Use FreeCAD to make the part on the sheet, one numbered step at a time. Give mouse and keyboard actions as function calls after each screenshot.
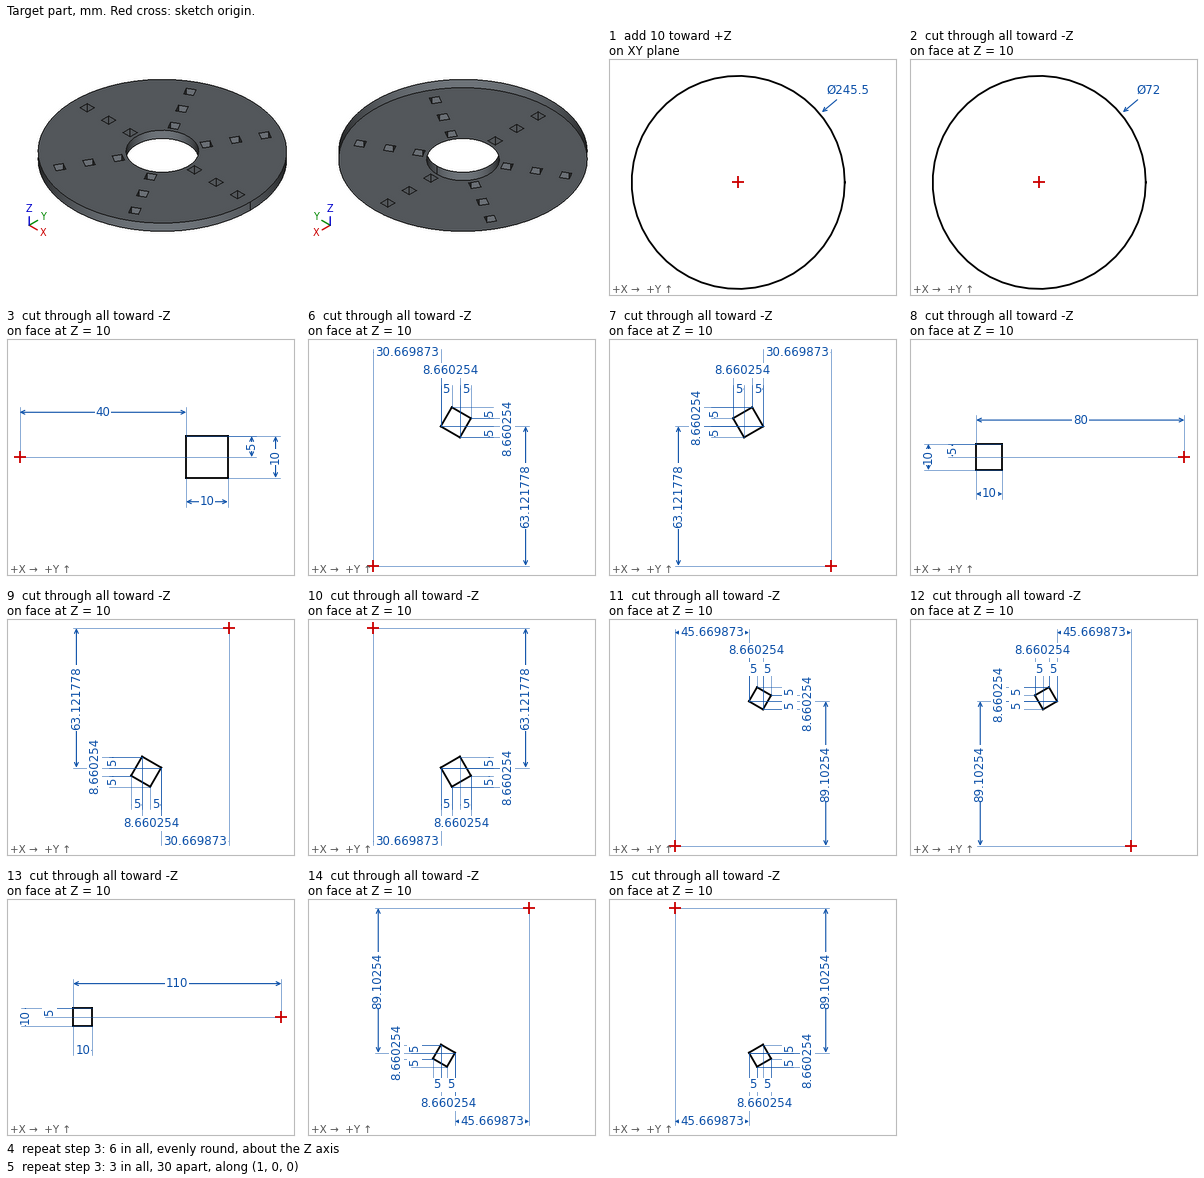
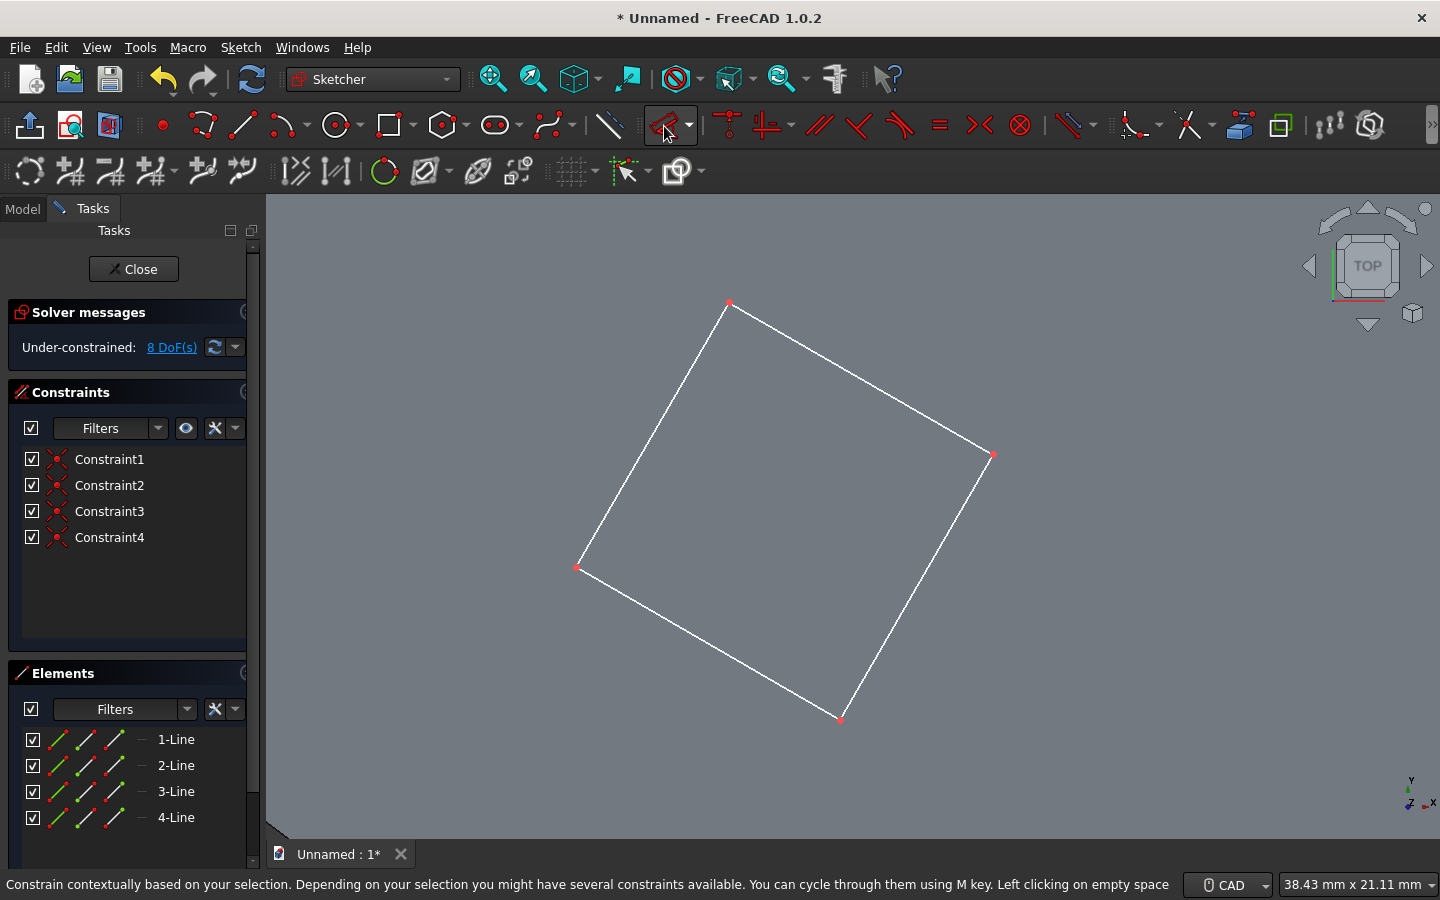
click(914, 409)
click(1027, 379)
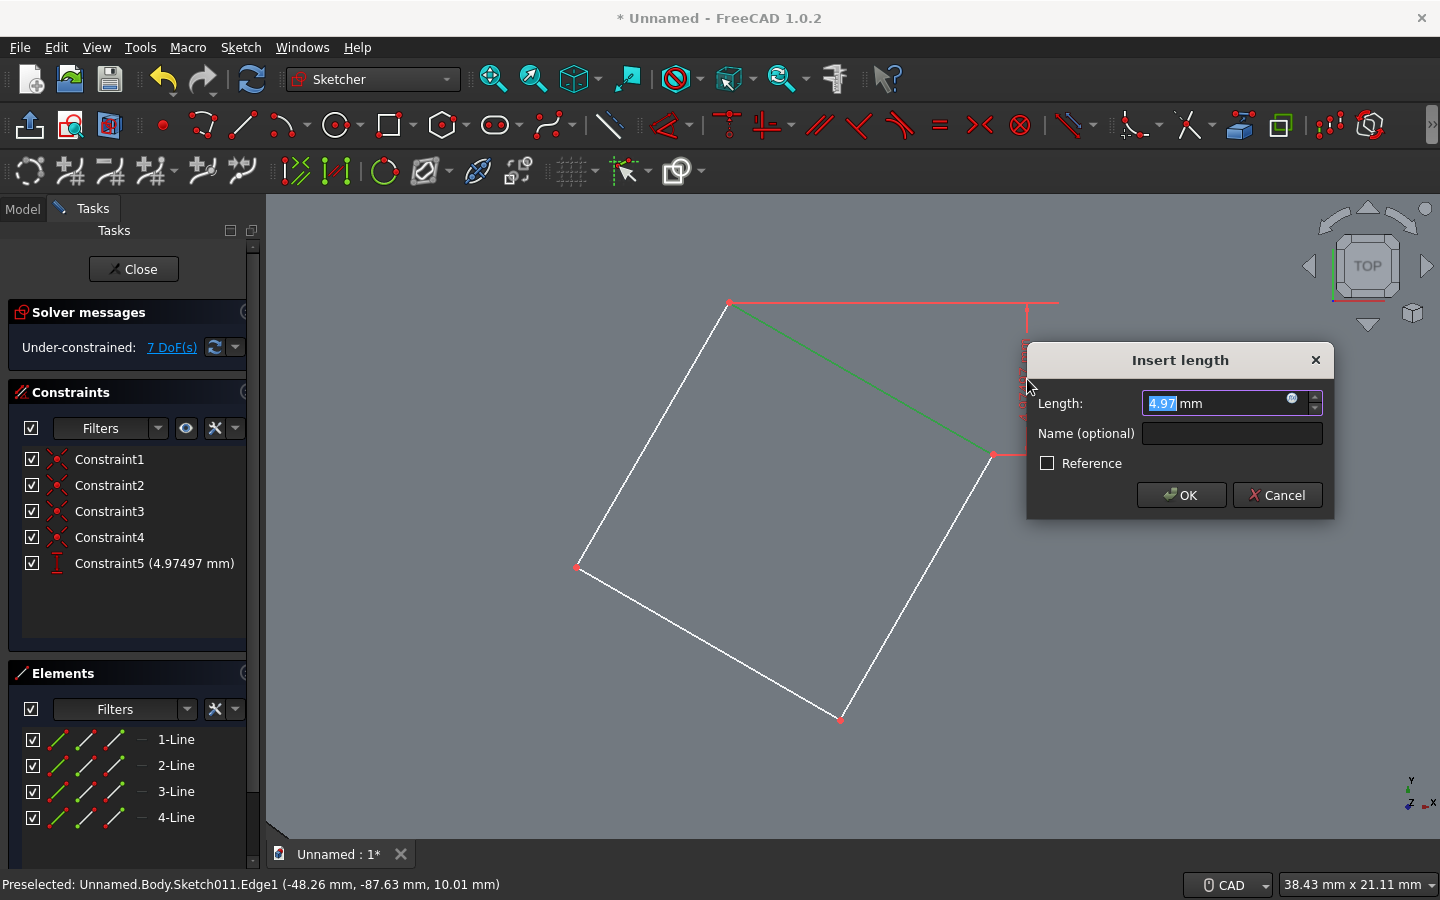
text(5)
key(Return)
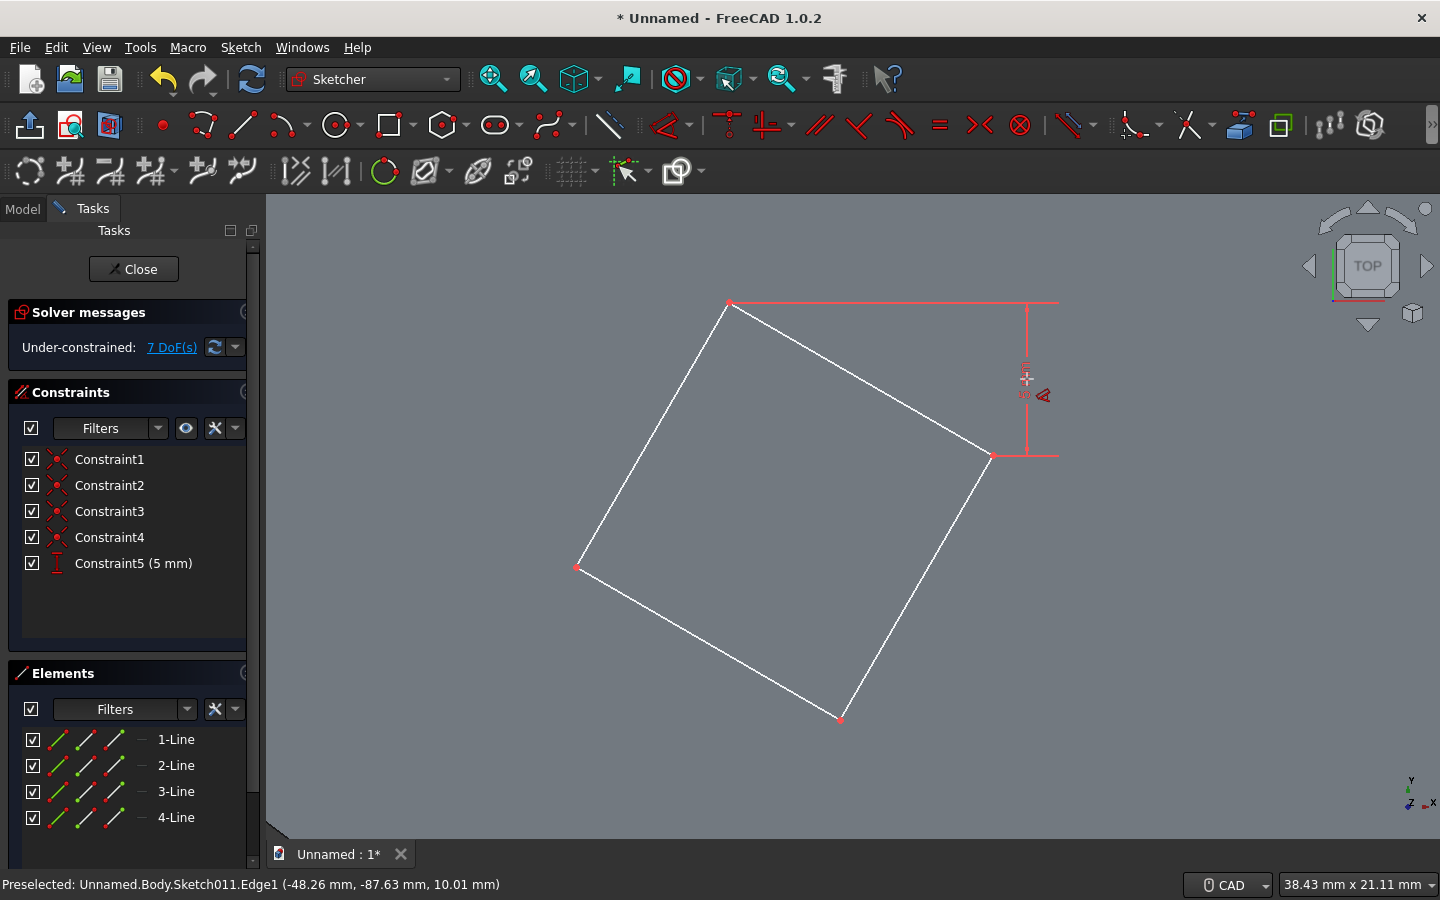
click(683, 382)
click(653, 269)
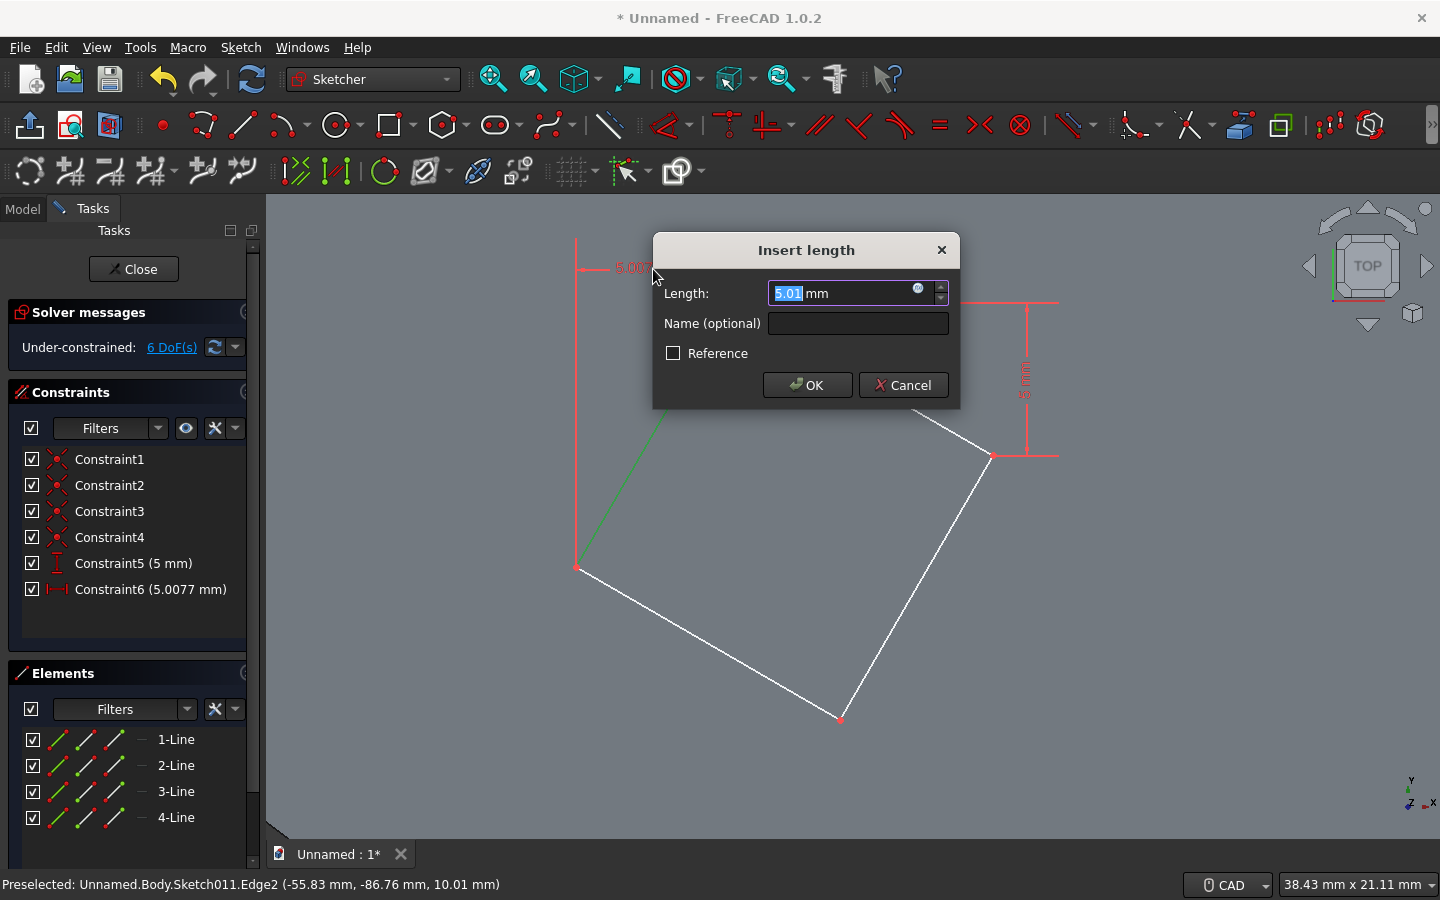
text(5)
key(Return)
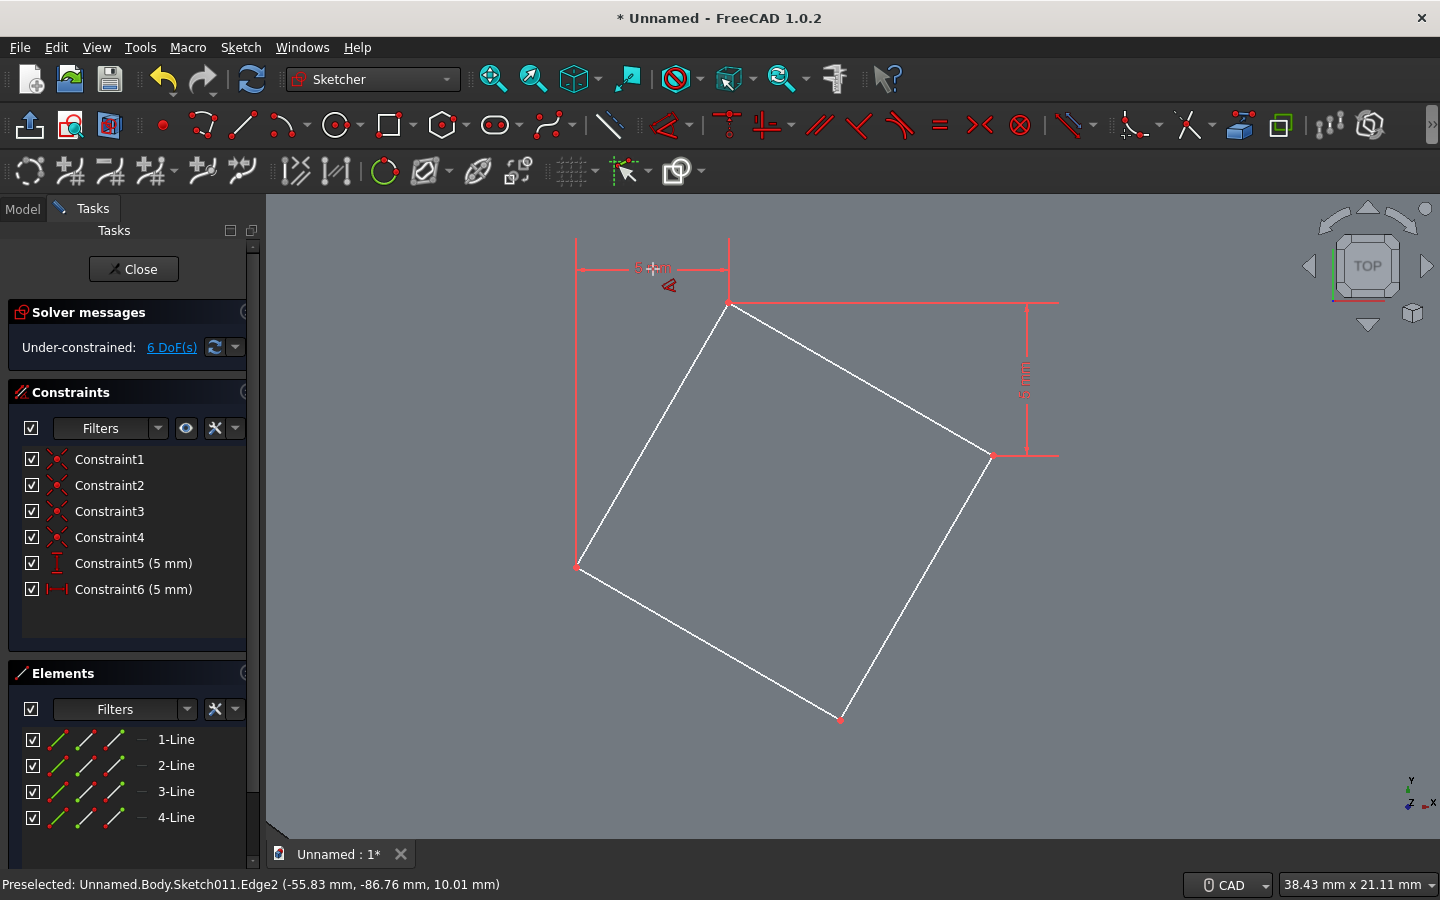
click(655, 613)
click(542, 644)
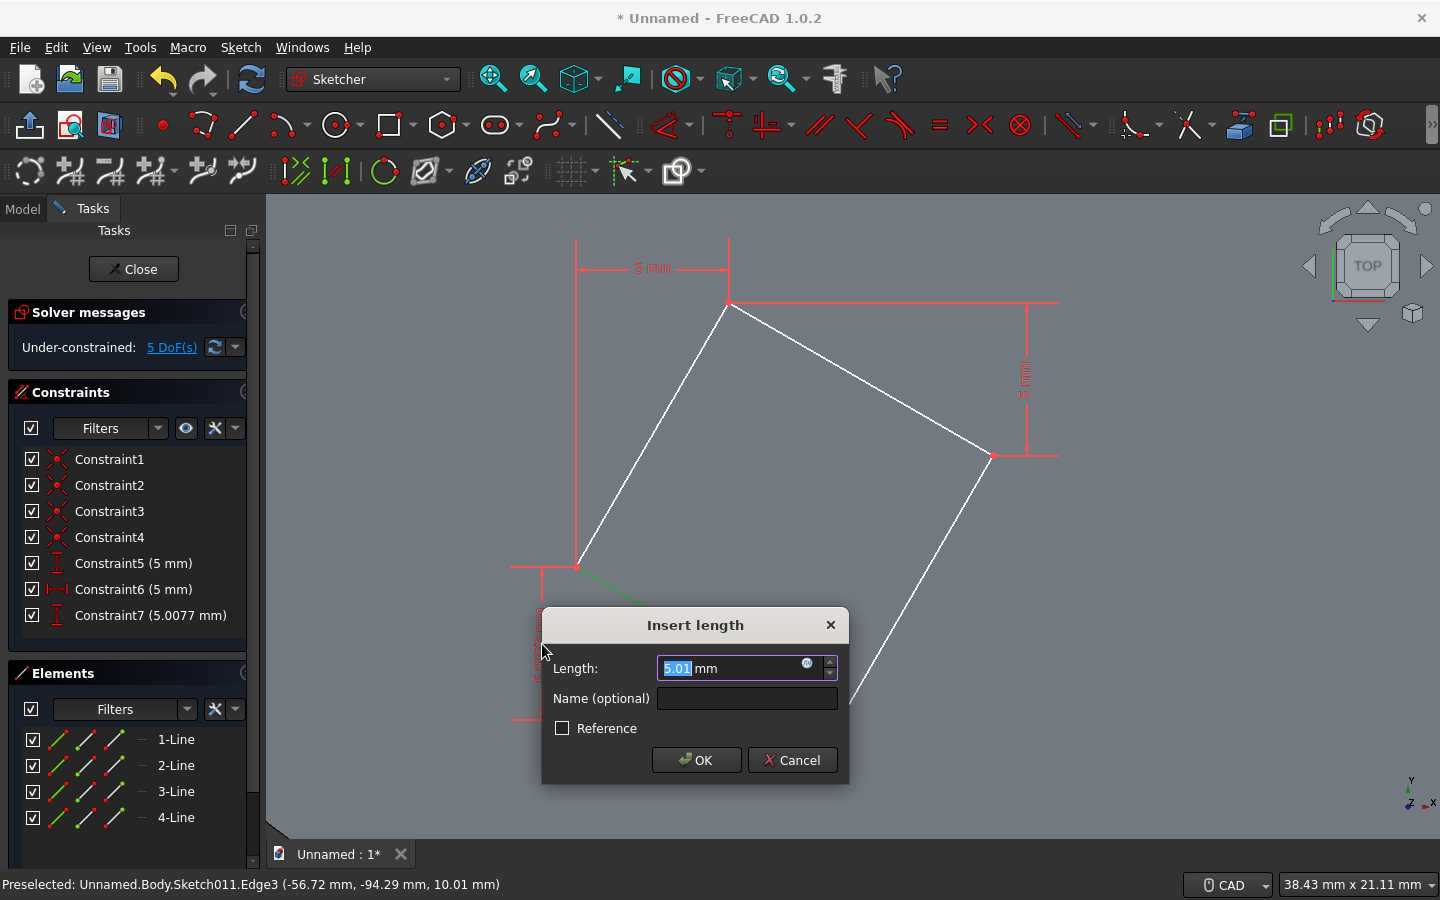
text(5)
key(Return)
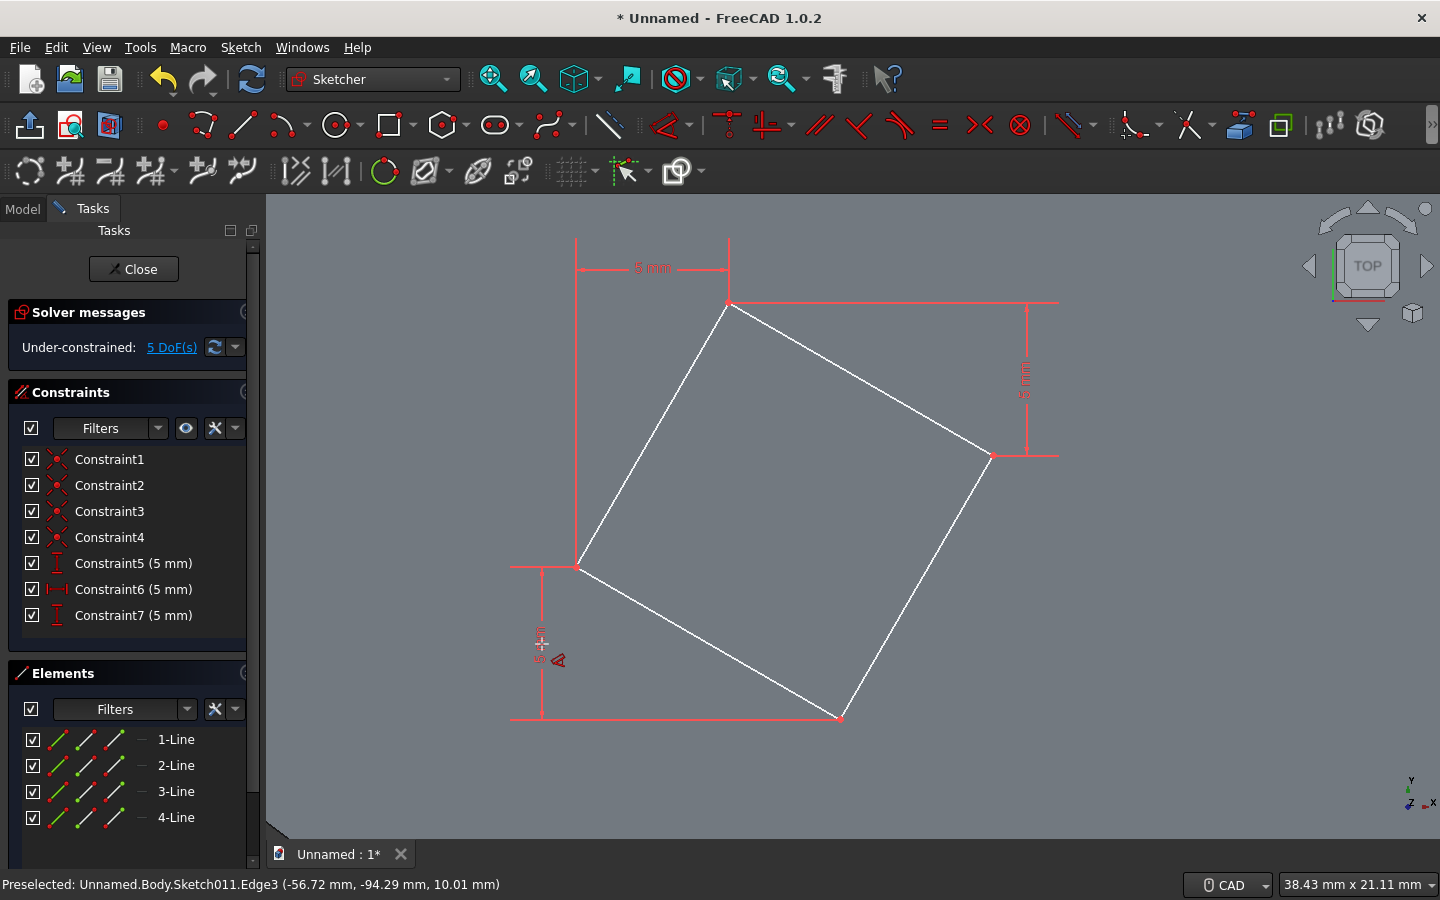
click(886, 641)
click(916, 754)